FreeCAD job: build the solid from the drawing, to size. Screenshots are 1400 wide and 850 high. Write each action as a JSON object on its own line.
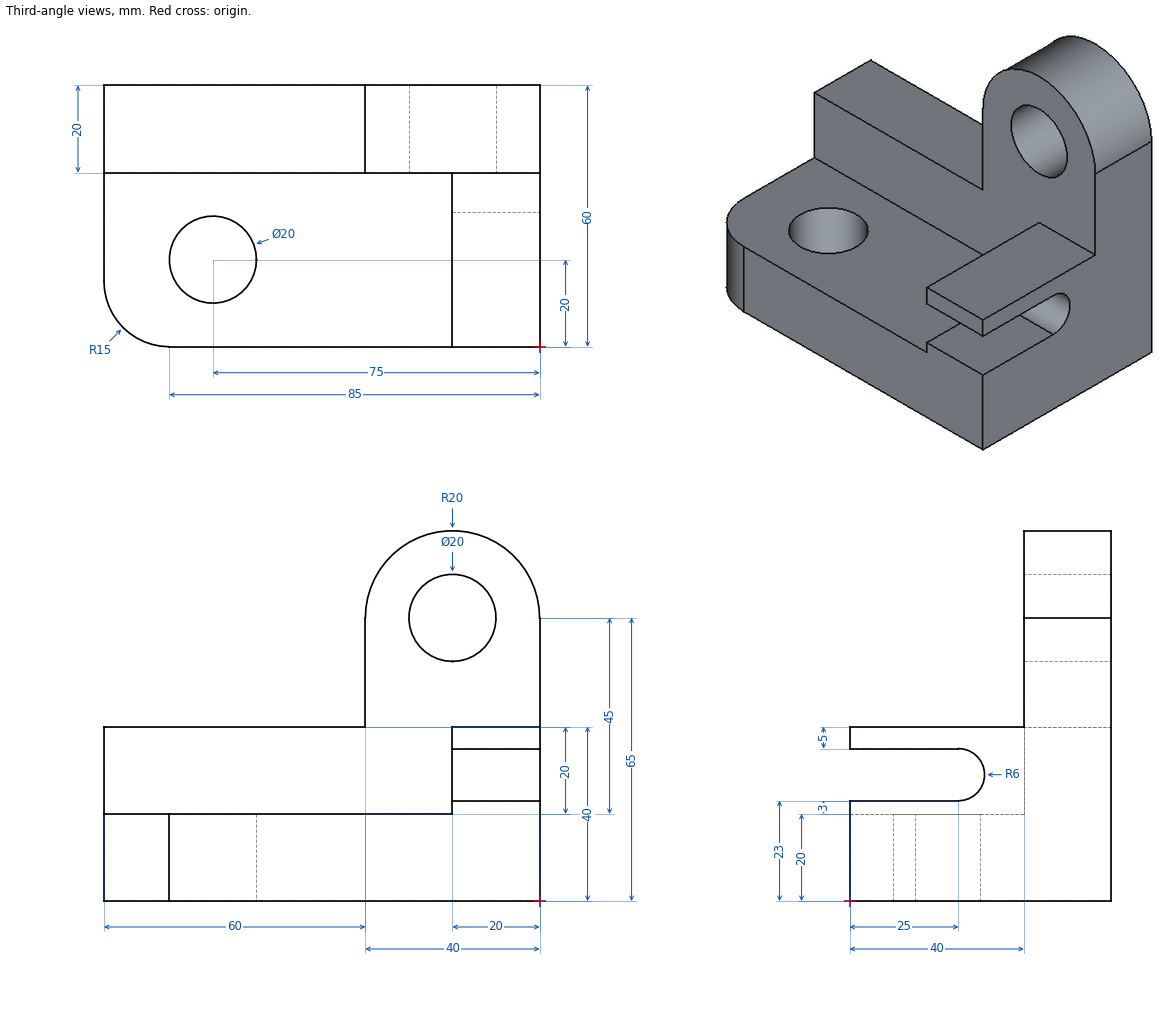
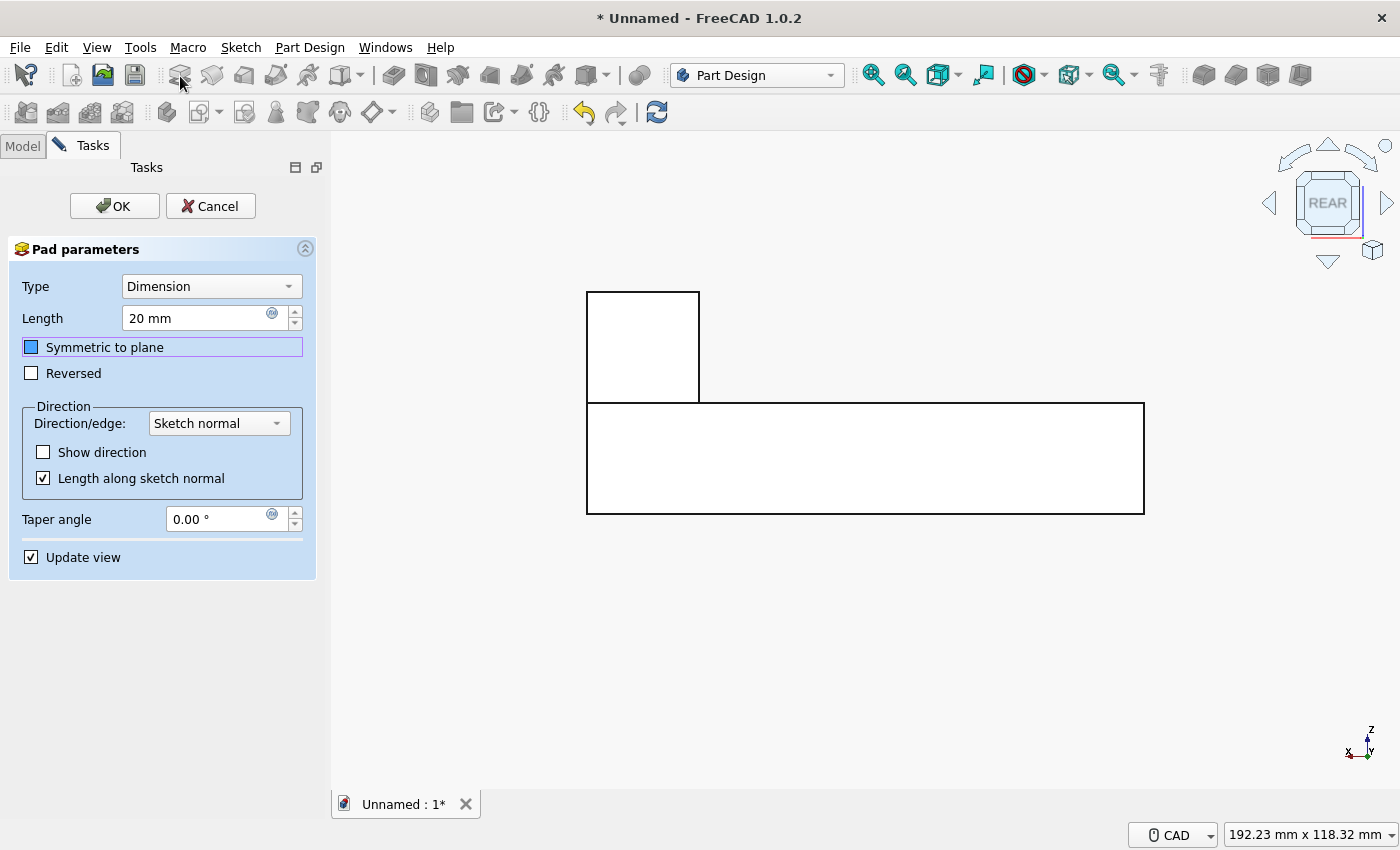
{"action": "left_click", "coordinate": [30, 373]}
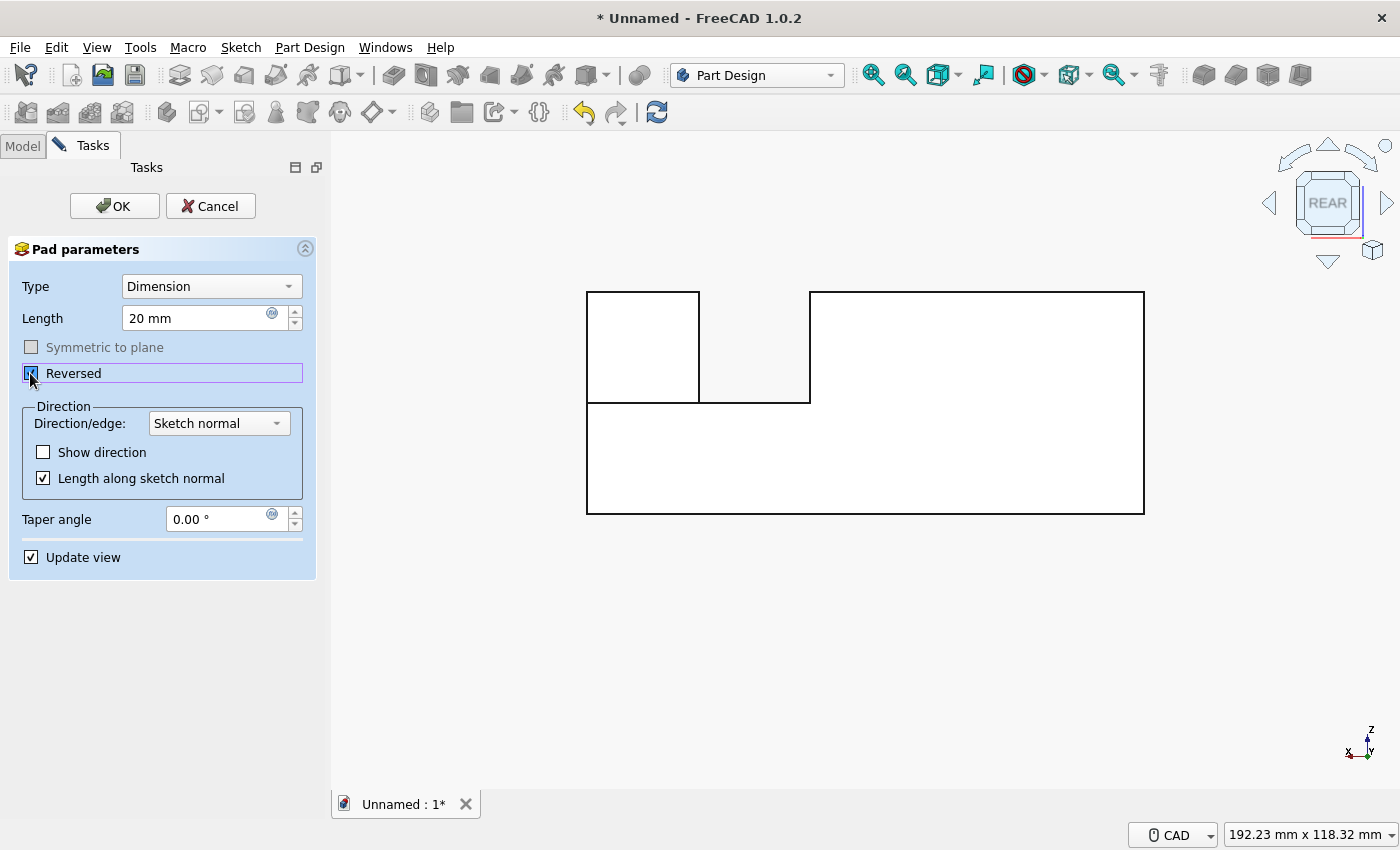
{"action": "left_click", "coordinate": [115, 206]}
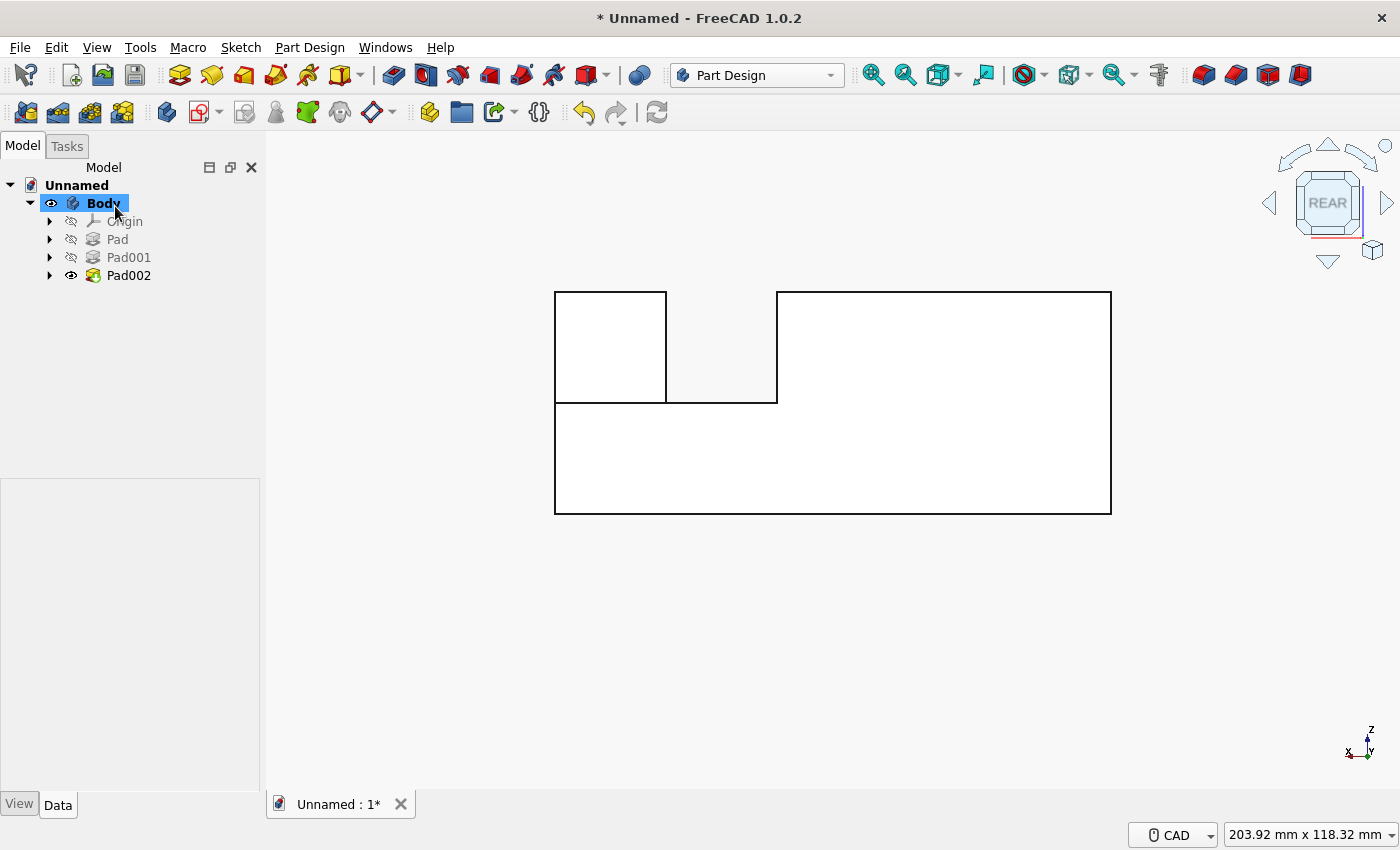
{"action": "left_click", "coordinate": [912, 402]}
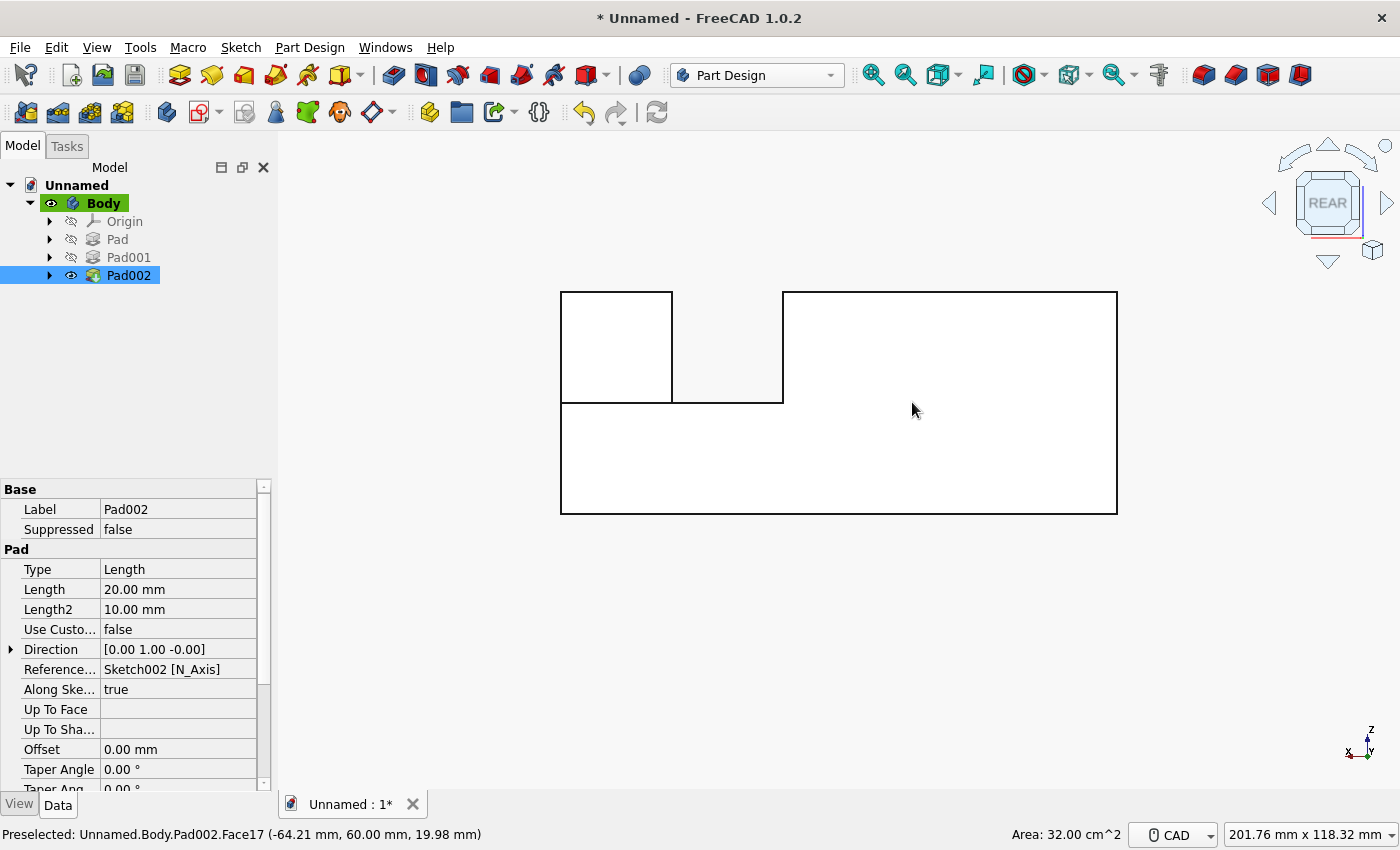
{"action": "left_click", "coordinate": [200, 112]}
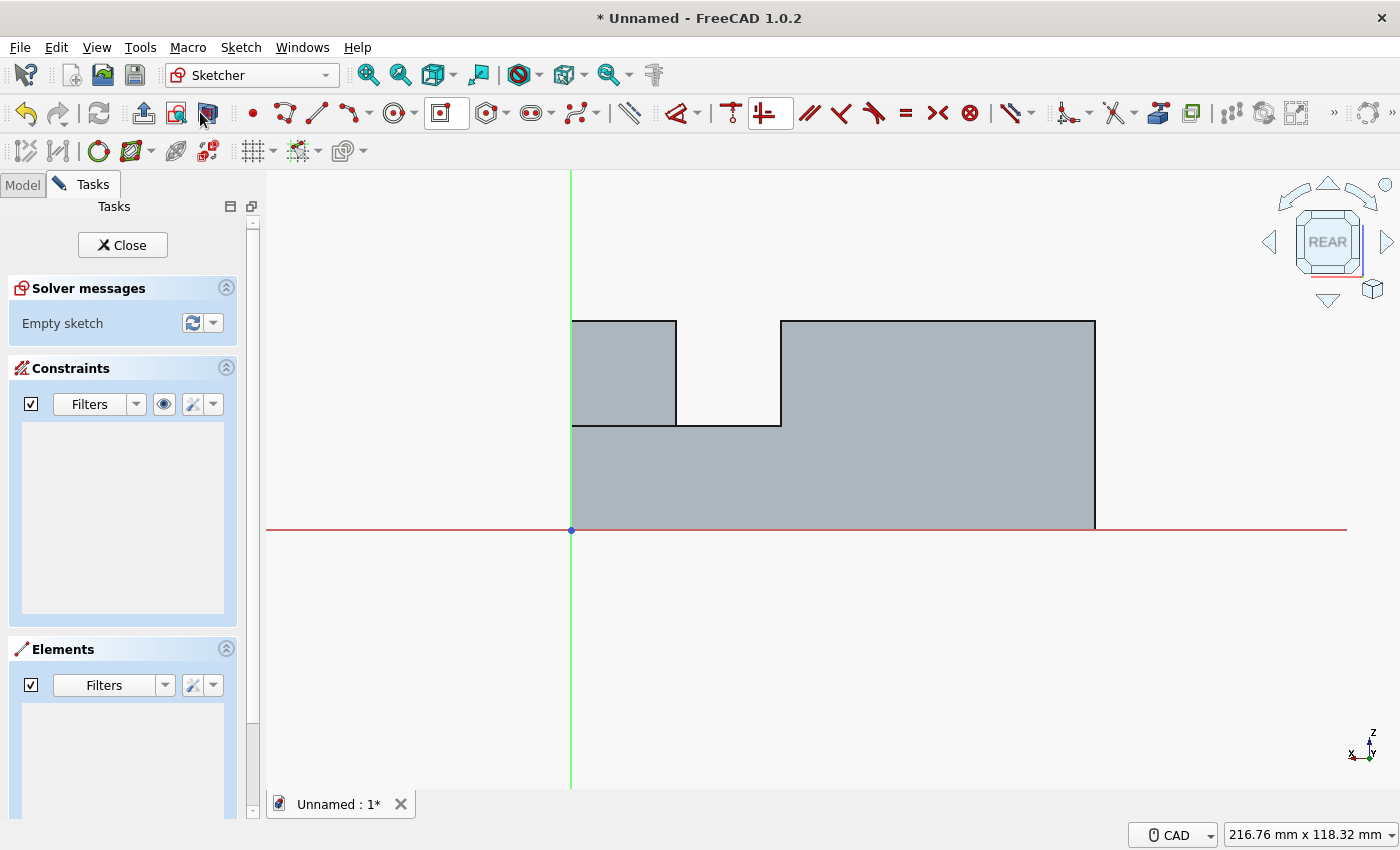
{"action": "scroll", "coordinate": [944, 761], "scroll_direction": "down", "scroll_amount": 2}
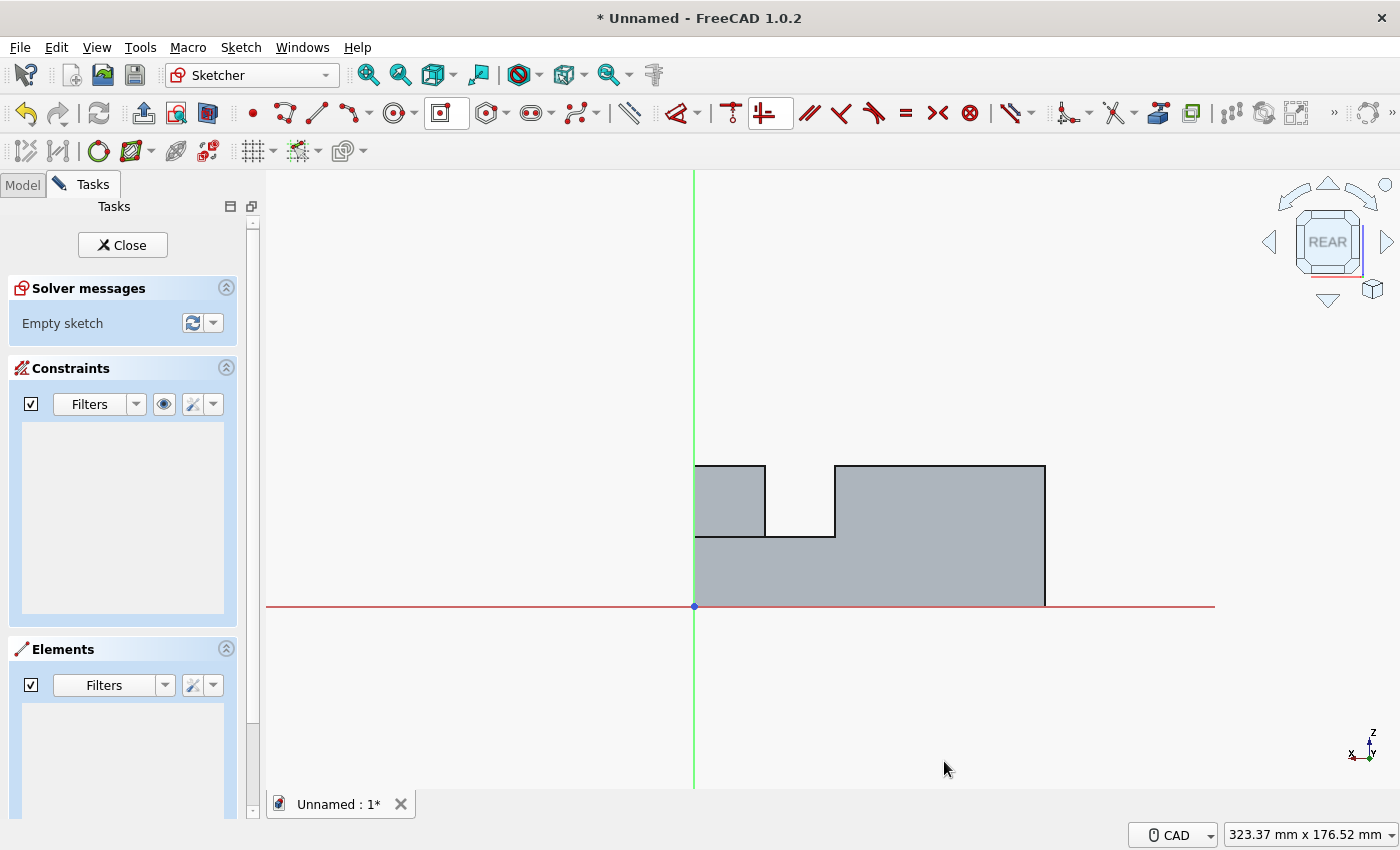
{"action": "key", "text": "g m"}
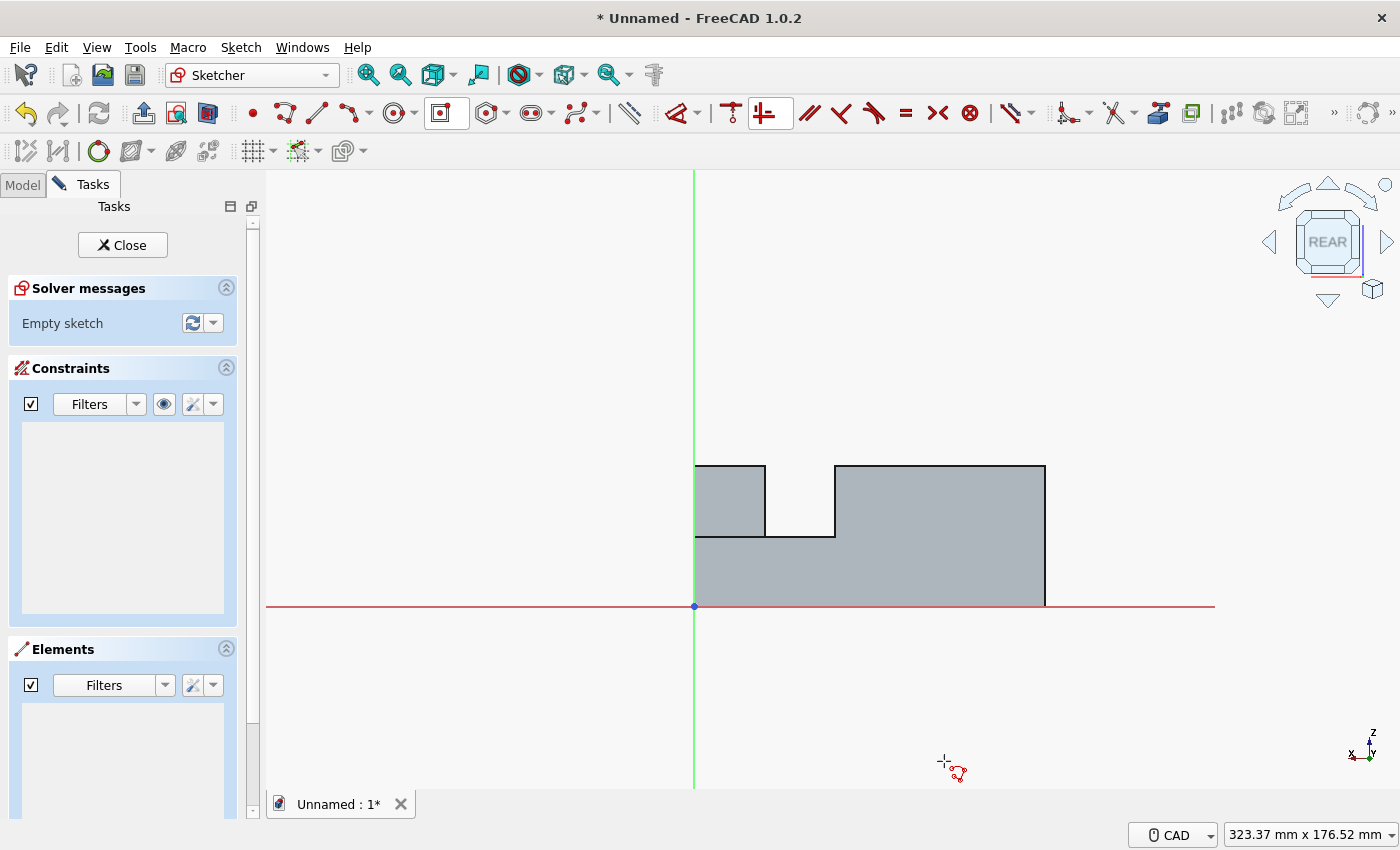
{"action": "left_click", "coordinate": [694, 379]}
{"action": "left_click", "coordinate": [703, 537]}
{"action": "left_click", "coordinate": [835, 537]}
{"action": "left_click", "coordinate": [835, 379]}
{"action": "right_click", "coordinate": [835, 379]}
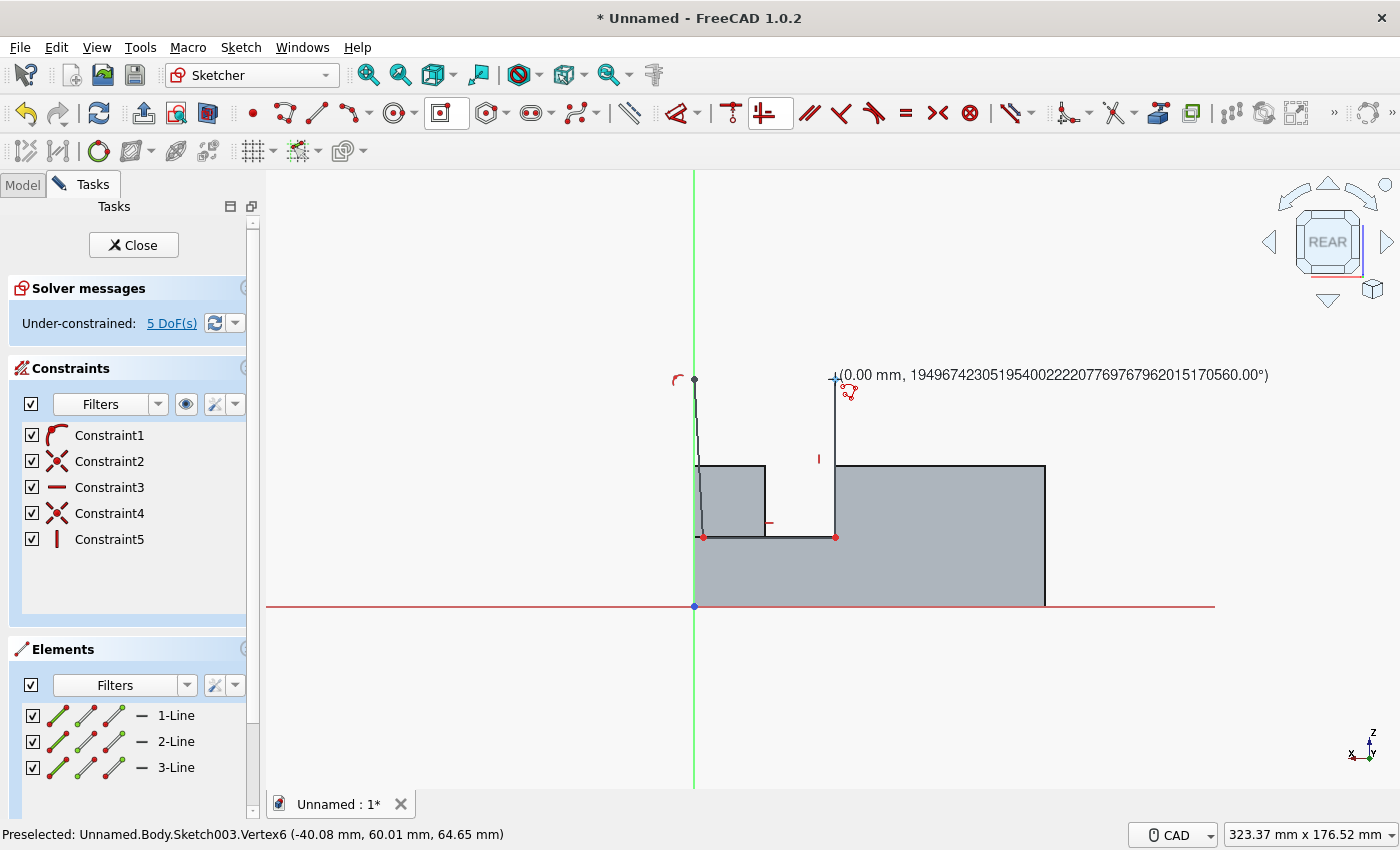
{"action": "key", "text": "g 3 a"}